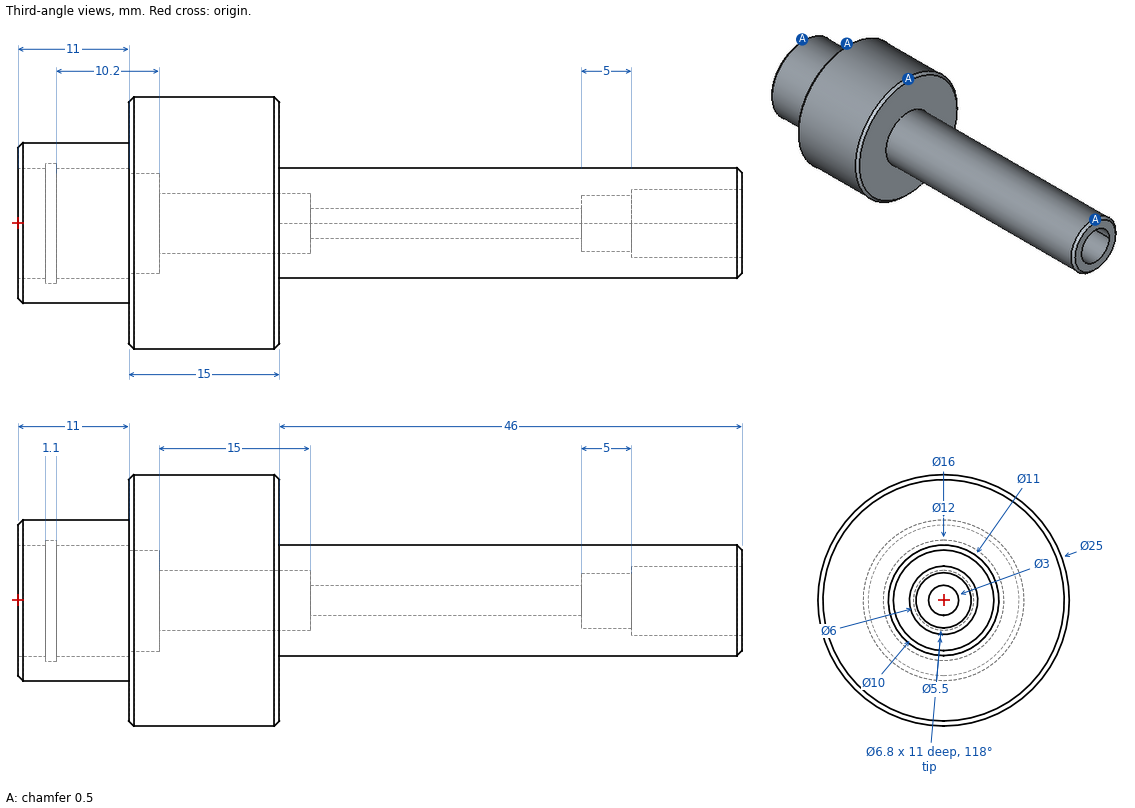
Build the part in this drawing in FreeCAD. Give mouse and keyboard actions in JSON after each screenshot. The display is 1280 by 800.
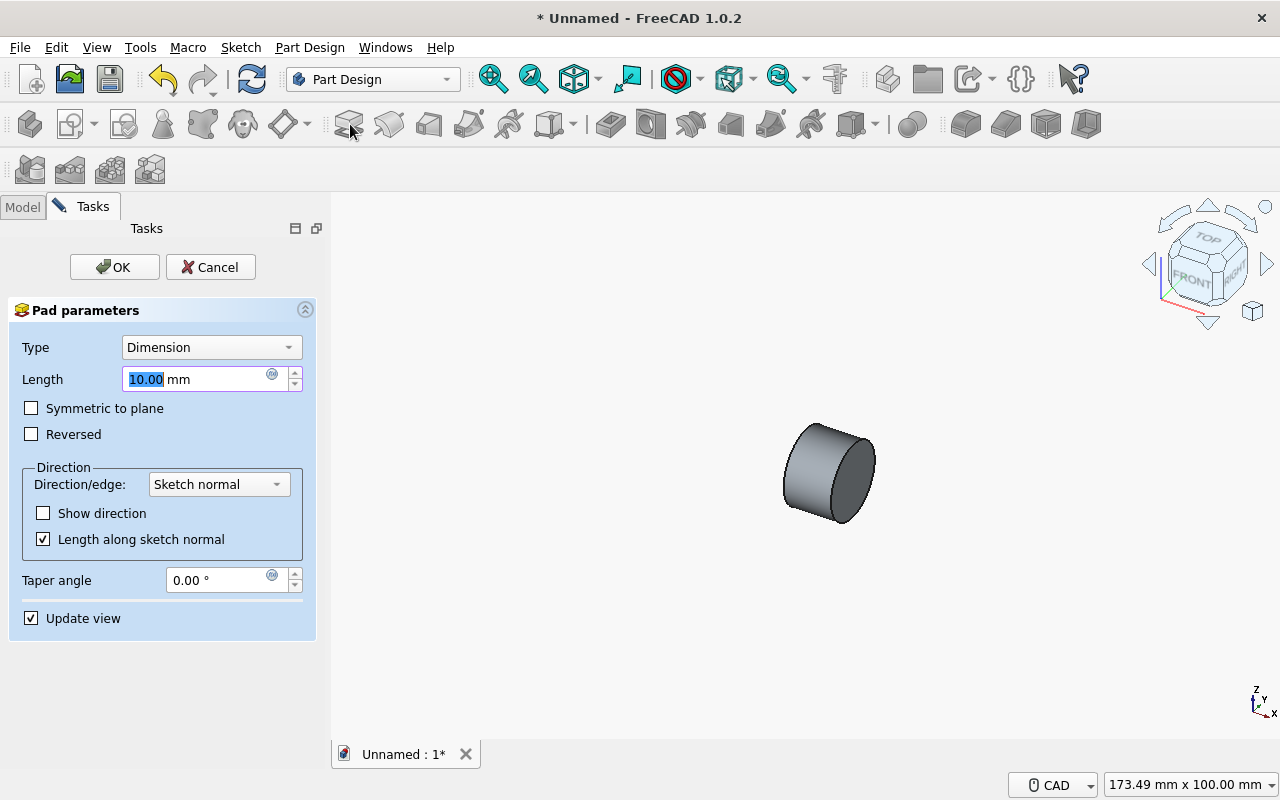
{"action": "type", "text": "11"}
{"action": "key", "text": "Tab"}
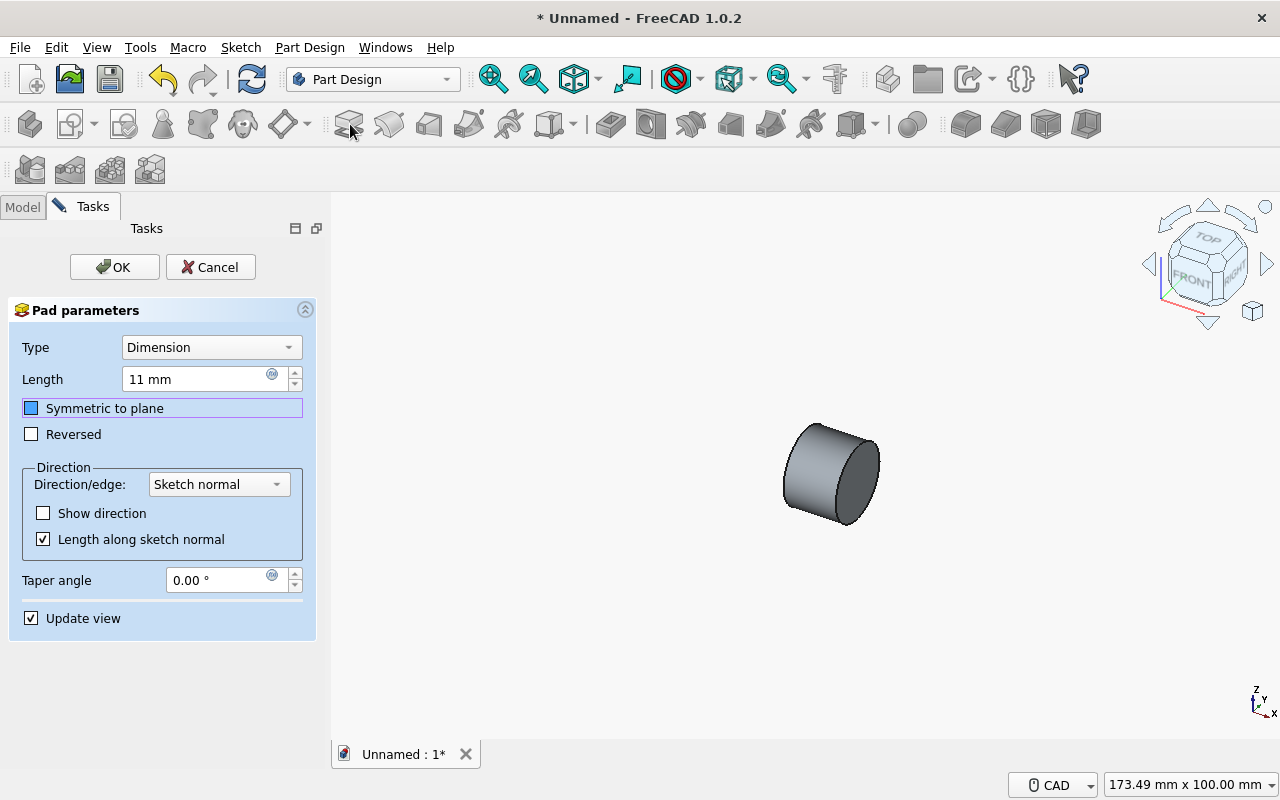
{"action": "left_click", "coordinate": [115, 267]}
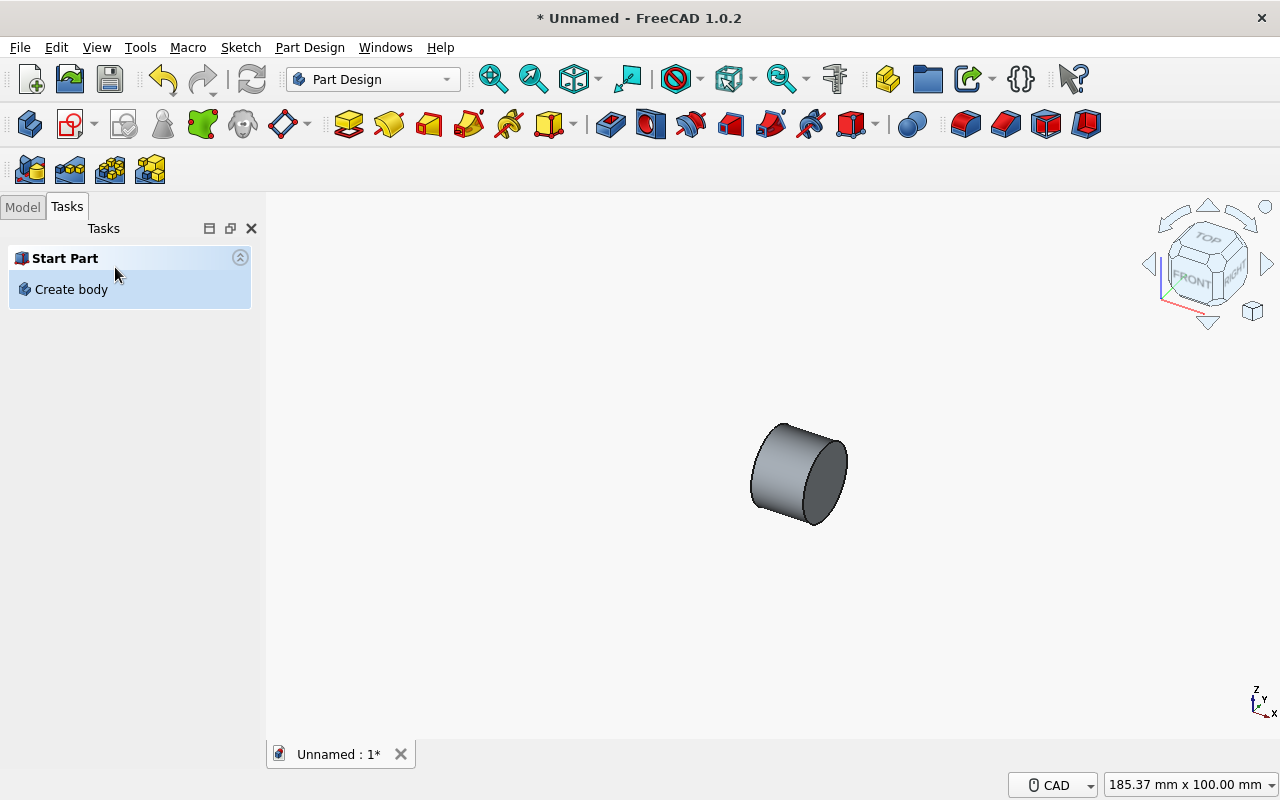
{"action": "key", "text": "v f"}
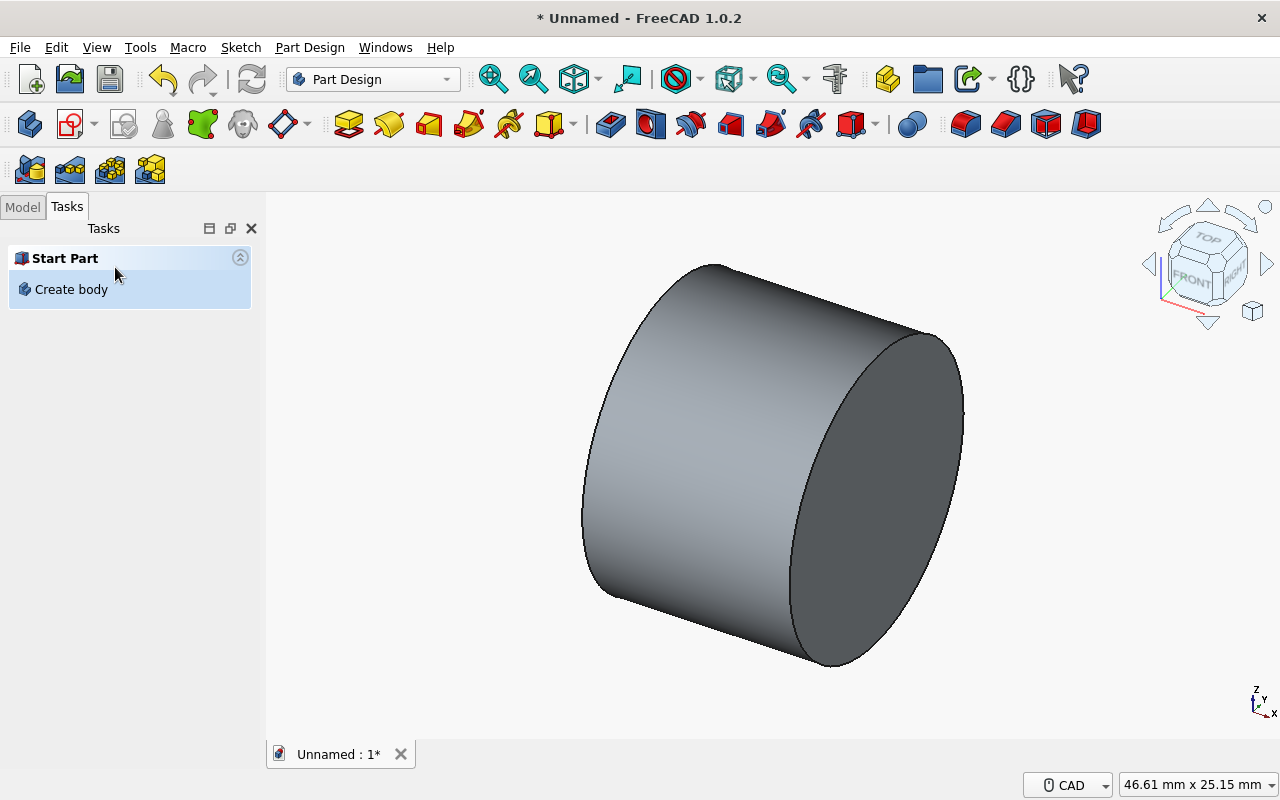
{"action": "left_click", "coordinate": [877, 499]}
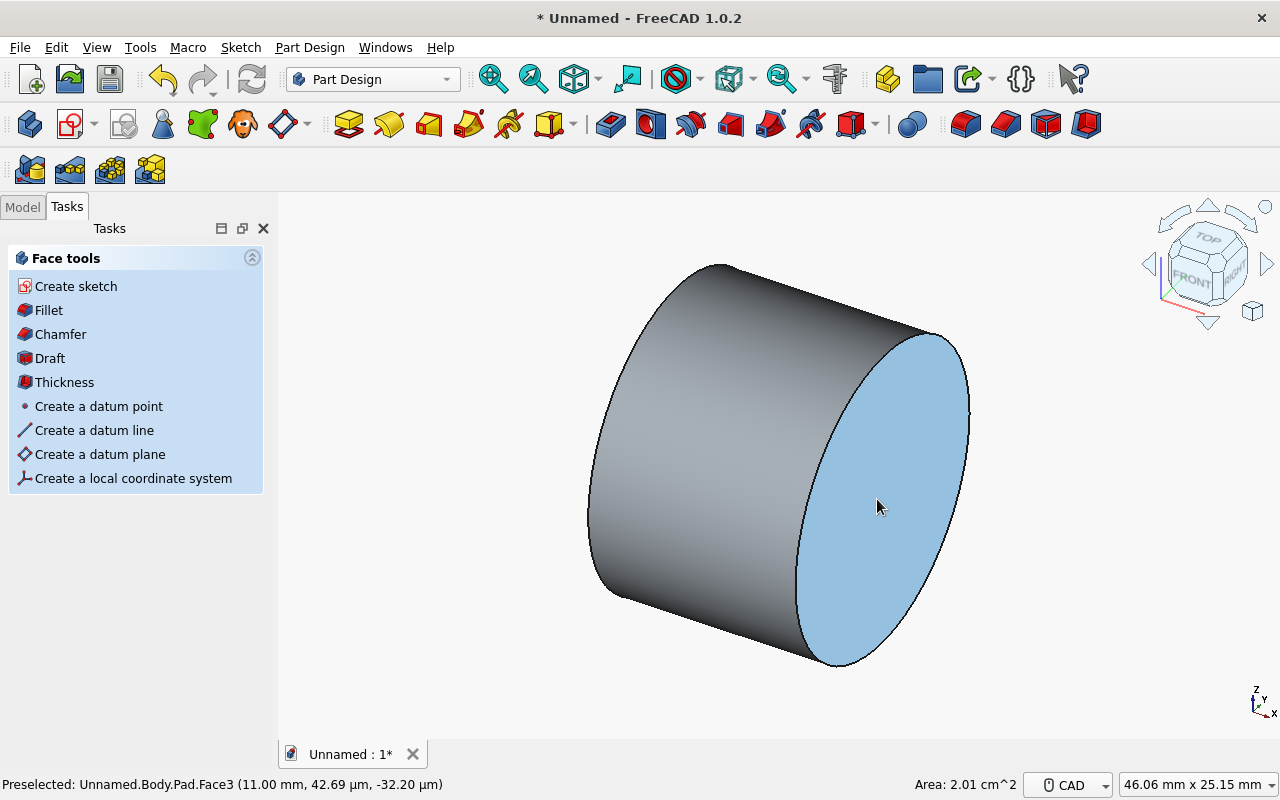
{"action": "left_click", "coordinate": [70, 124]}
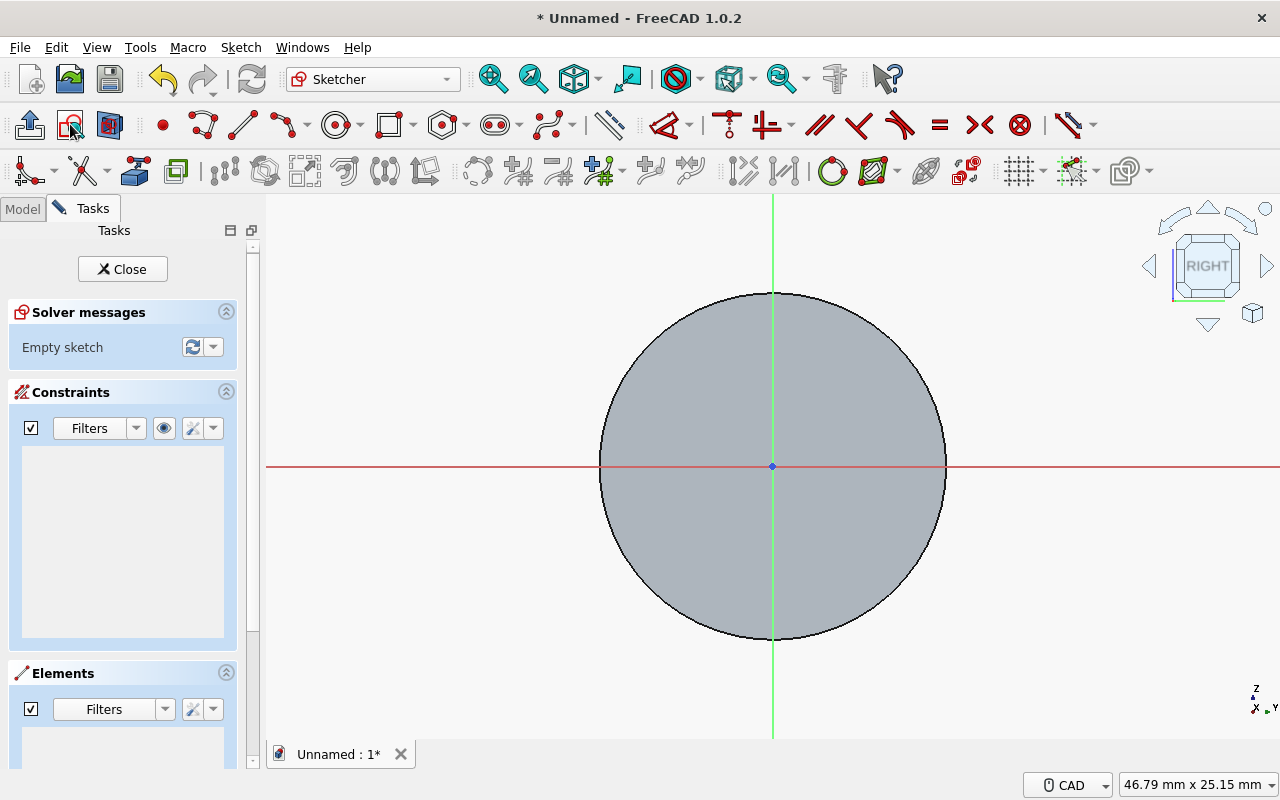
{"action": "scroll", "coordinate": [566, 466], "scroll_direction": "down", "scroll_amount": 2}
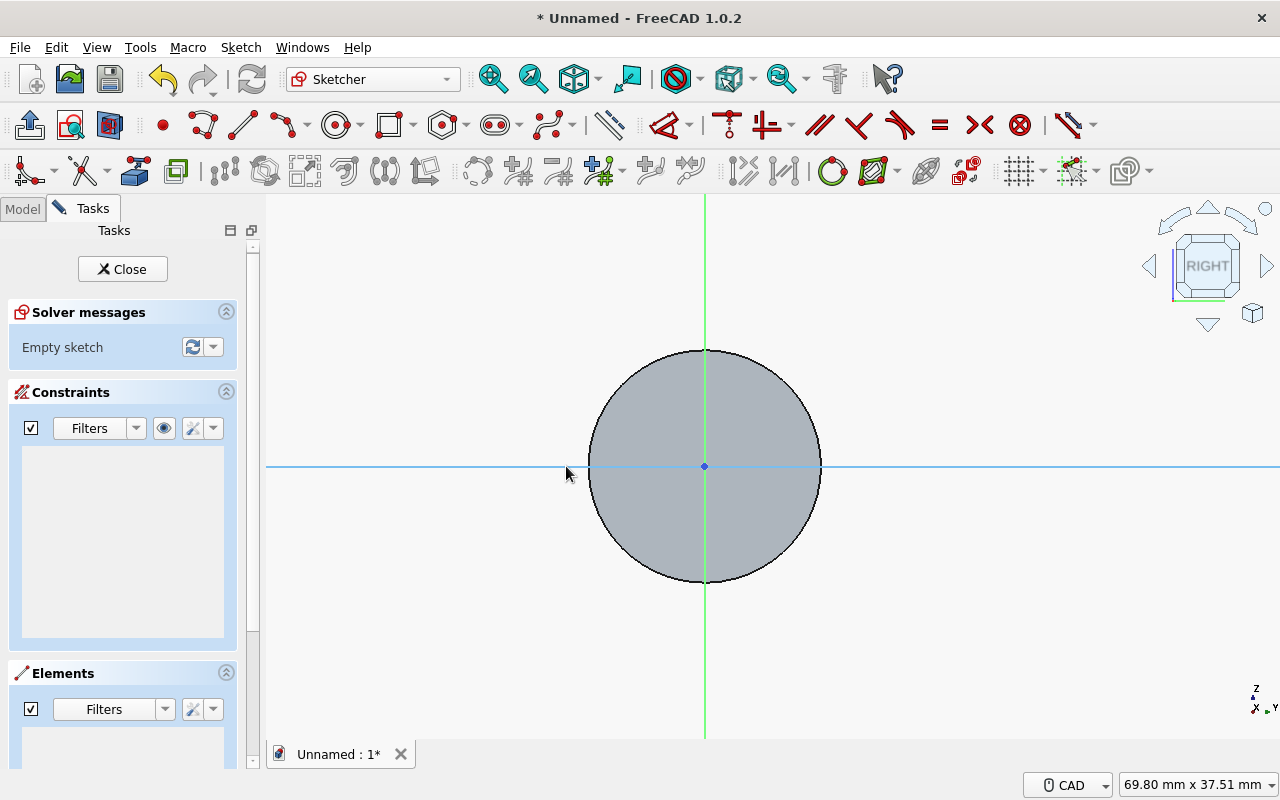
{"action": "left_click", "coordinate": [336, 126]}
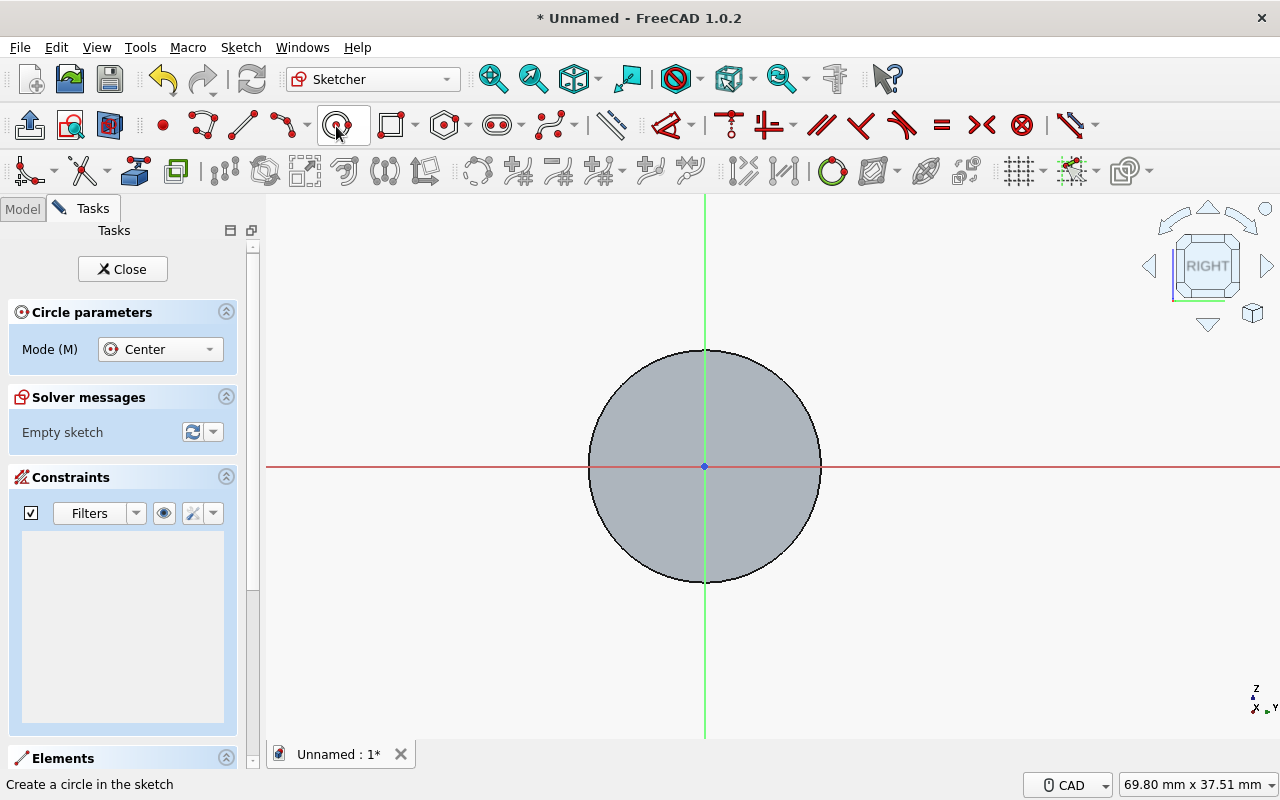
{"action": "left_click", "coordinate": [705, 466]}
{"action": "mouse_move", "coordinate": [833, 338]}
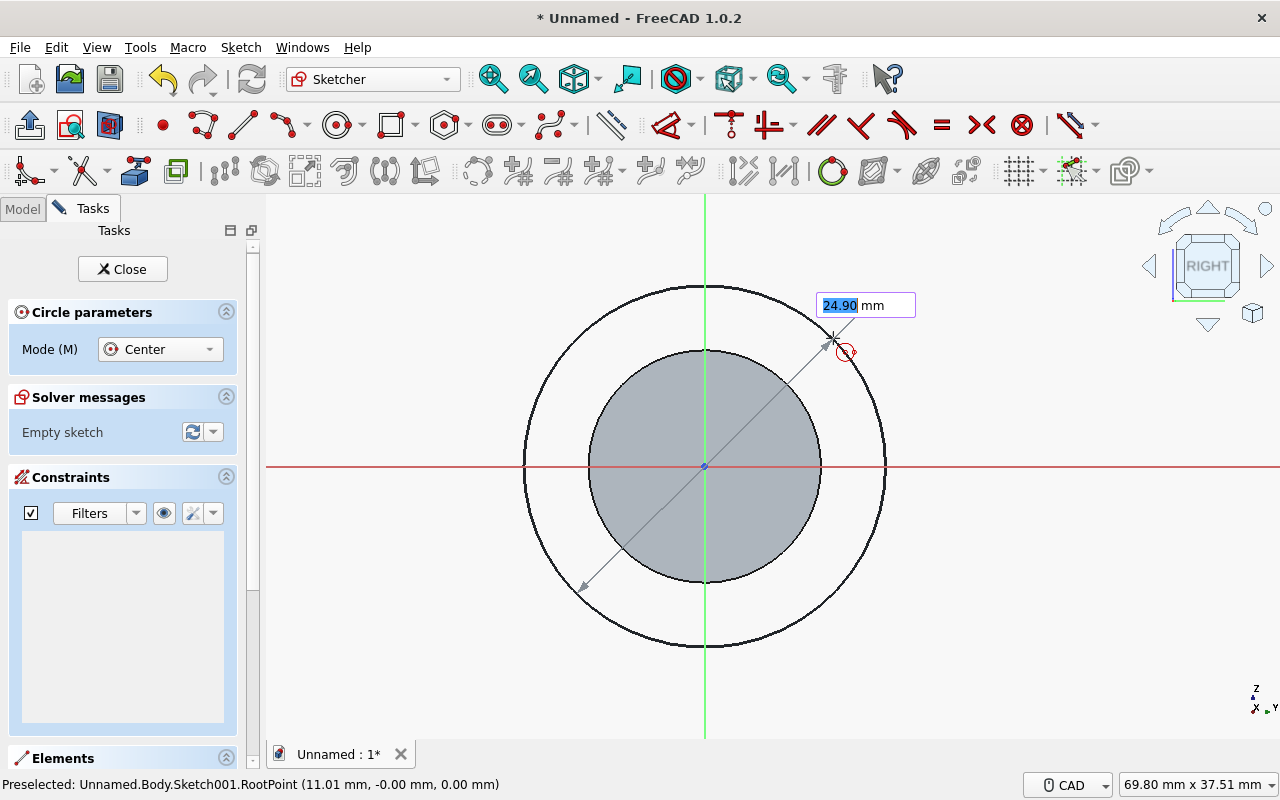
{"action": "type", "text": "25"}
{"action": "key", "text": "Return"}
{"action": "key", "text": "Escape"}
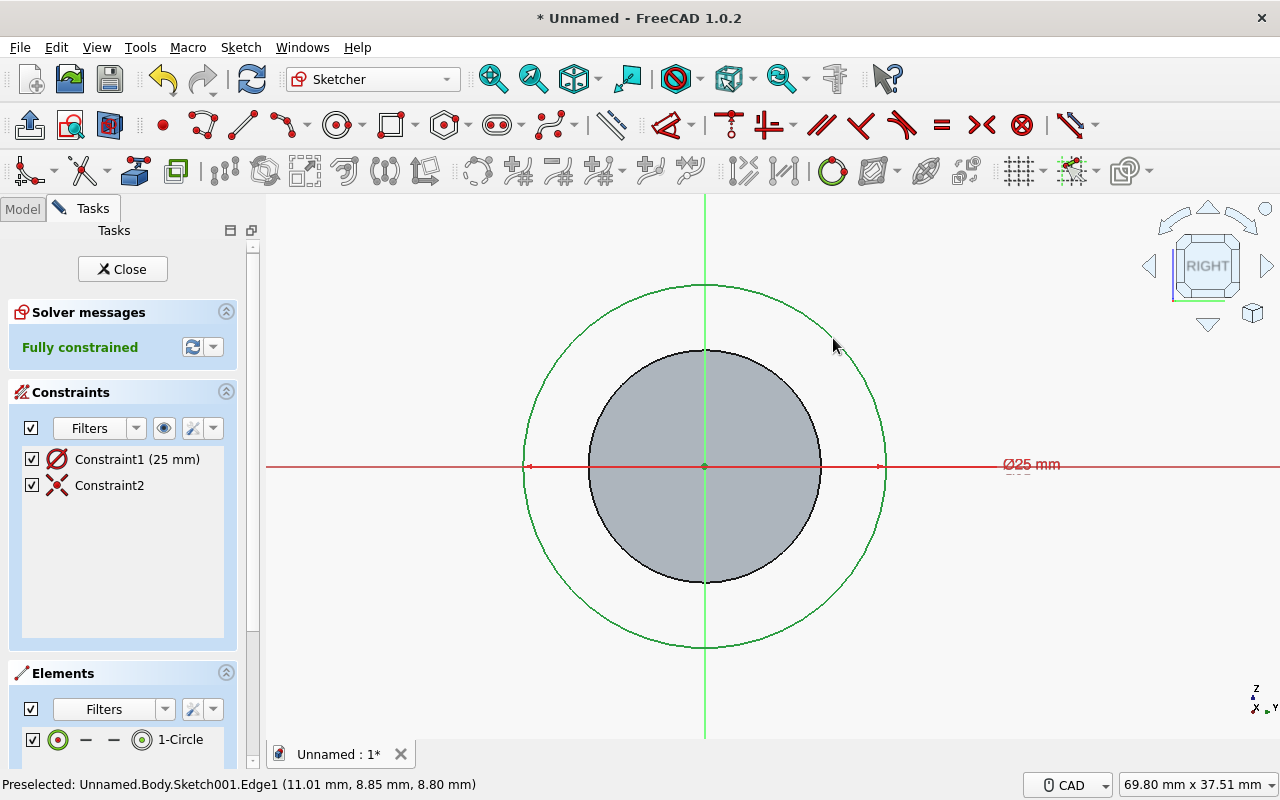
{"action": "left_click", "coordinate": [123, 269]}